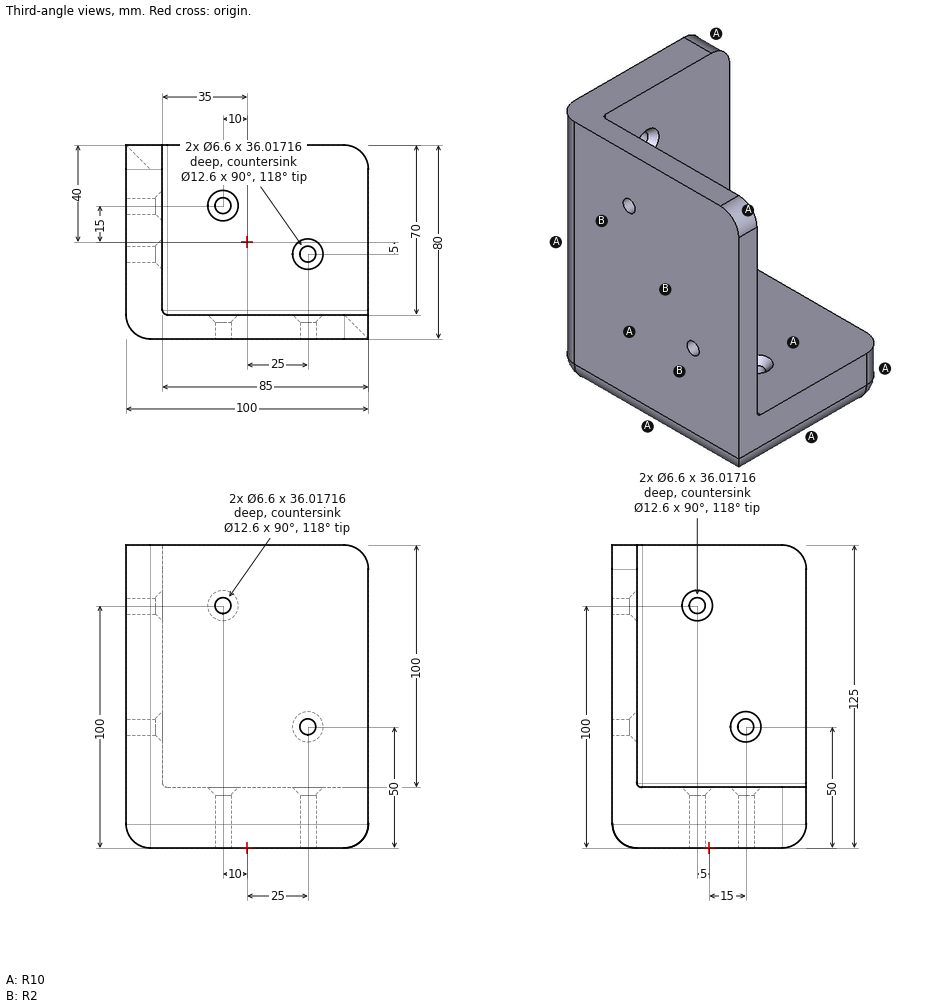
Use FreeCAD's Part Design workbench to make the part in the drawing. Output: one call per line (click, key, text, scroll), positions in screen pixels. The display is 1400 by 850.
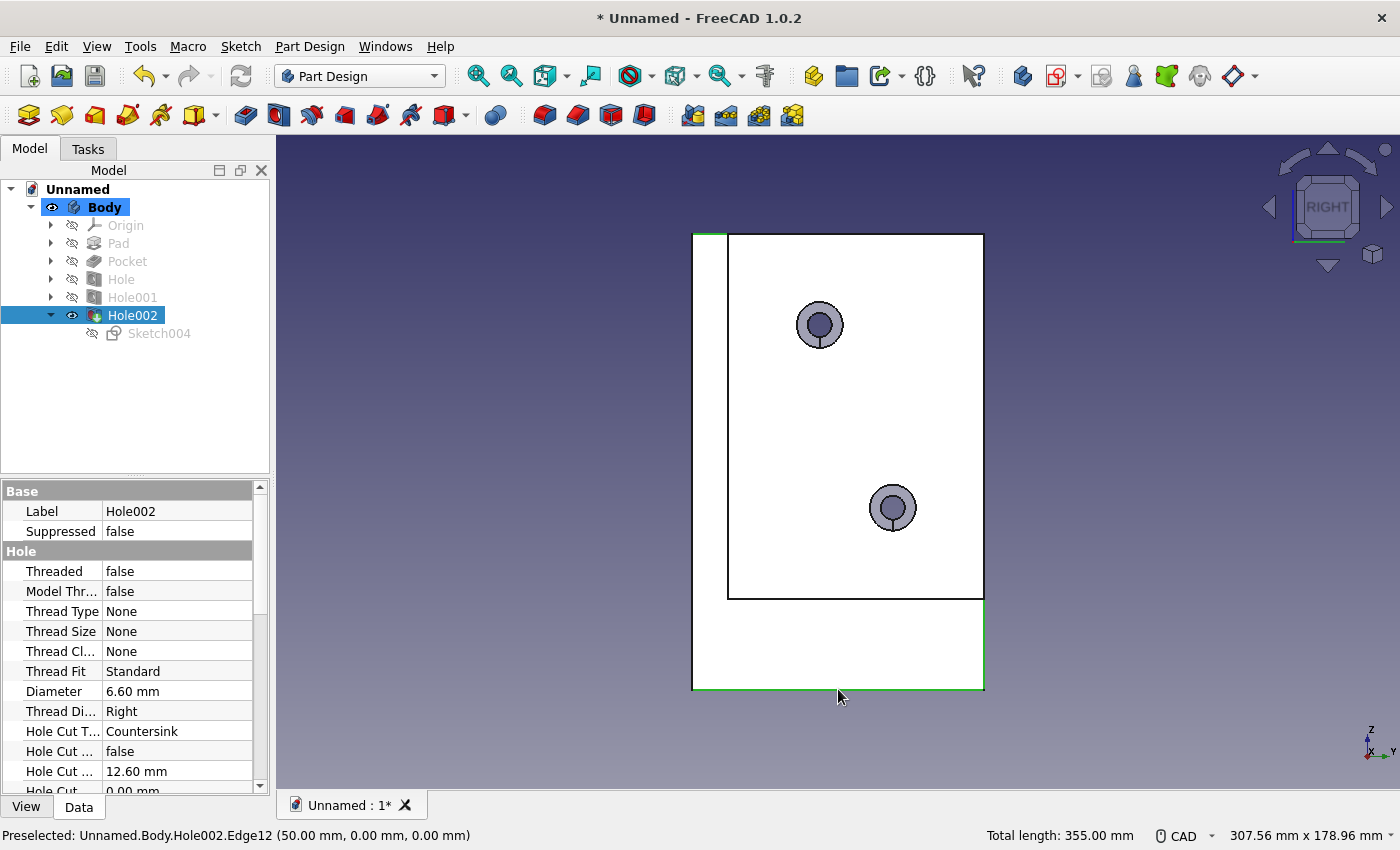
key(5)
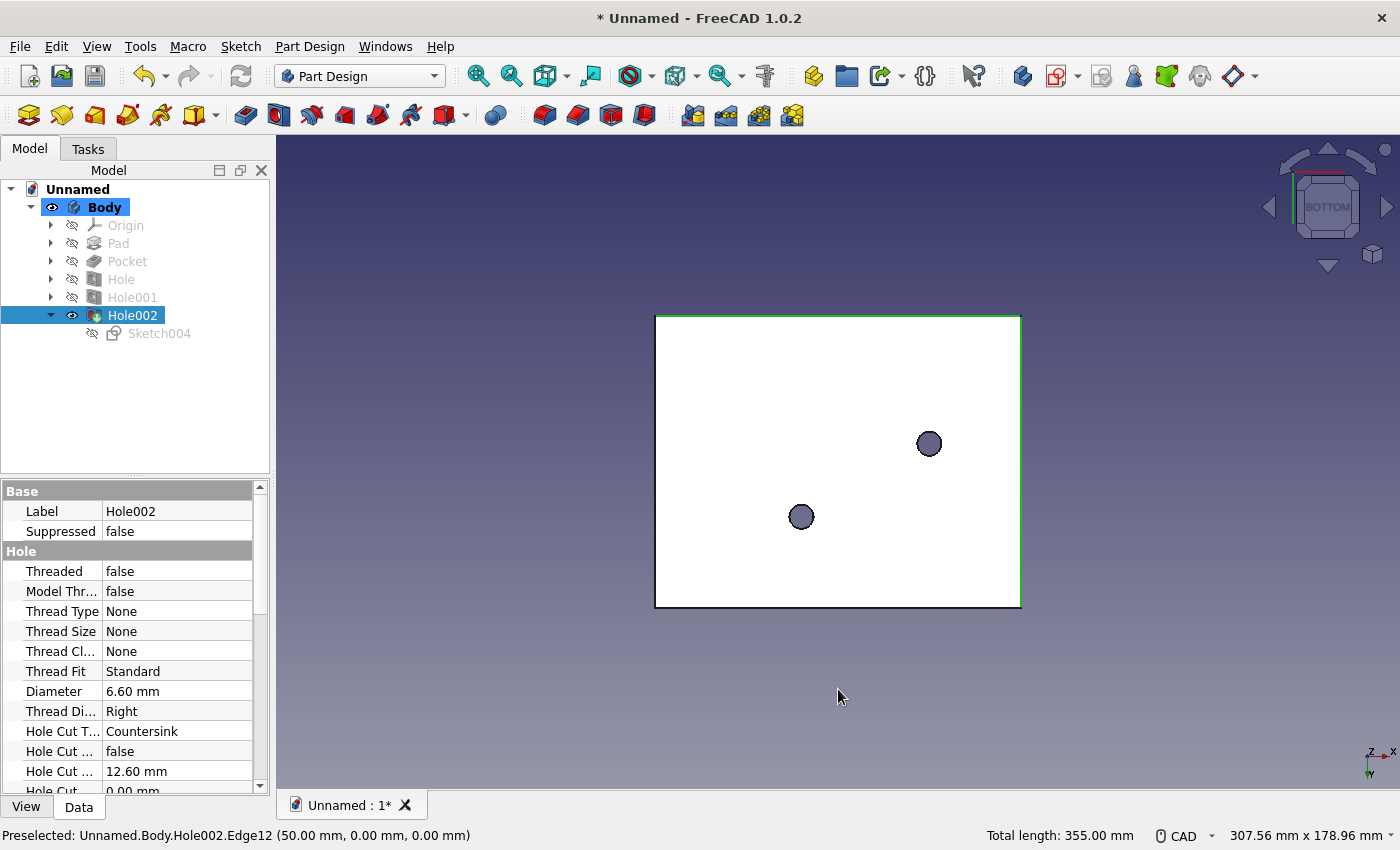
click(479, 76)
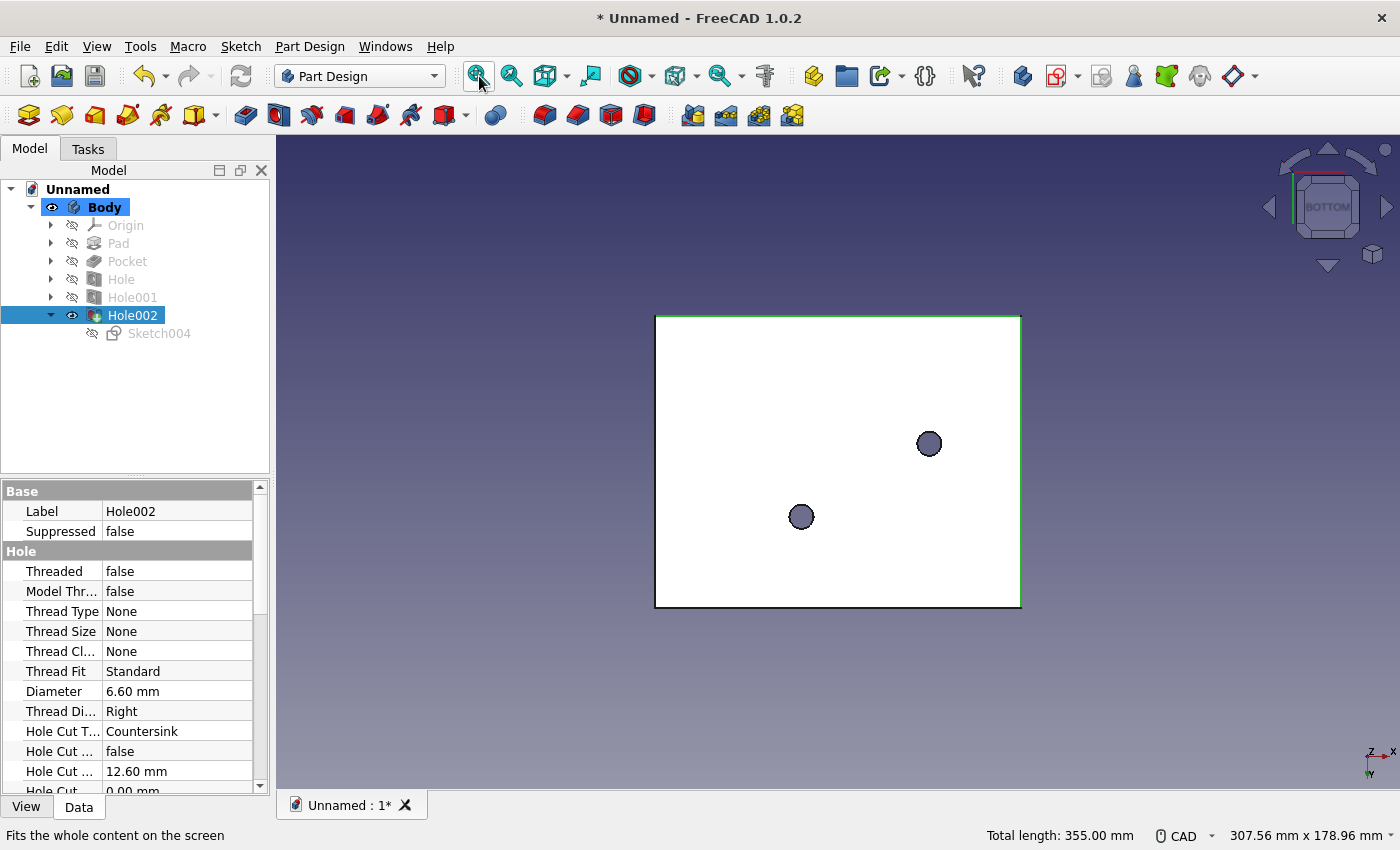
click(838, 607, ctrl)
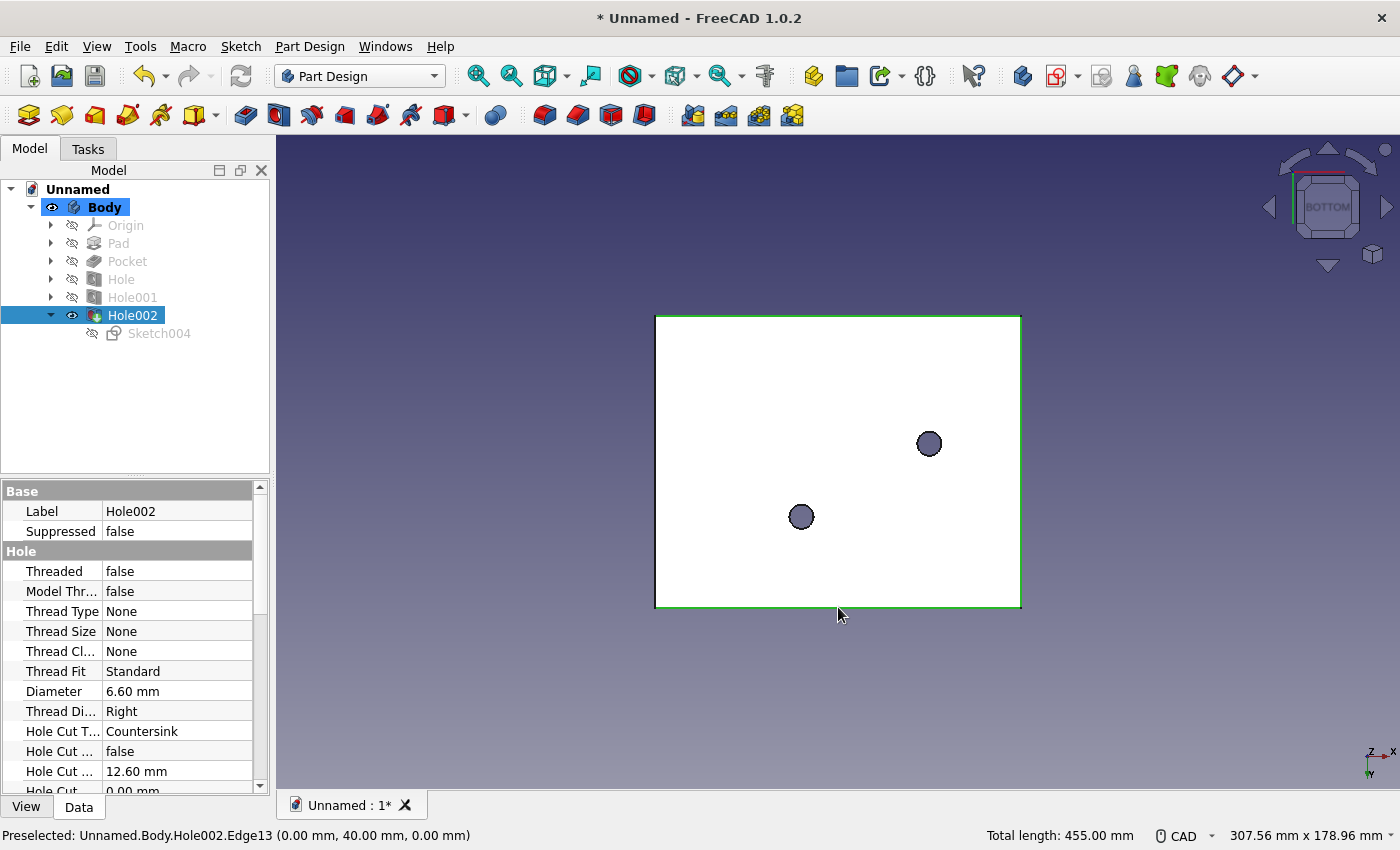
click(655, 461, ctrl)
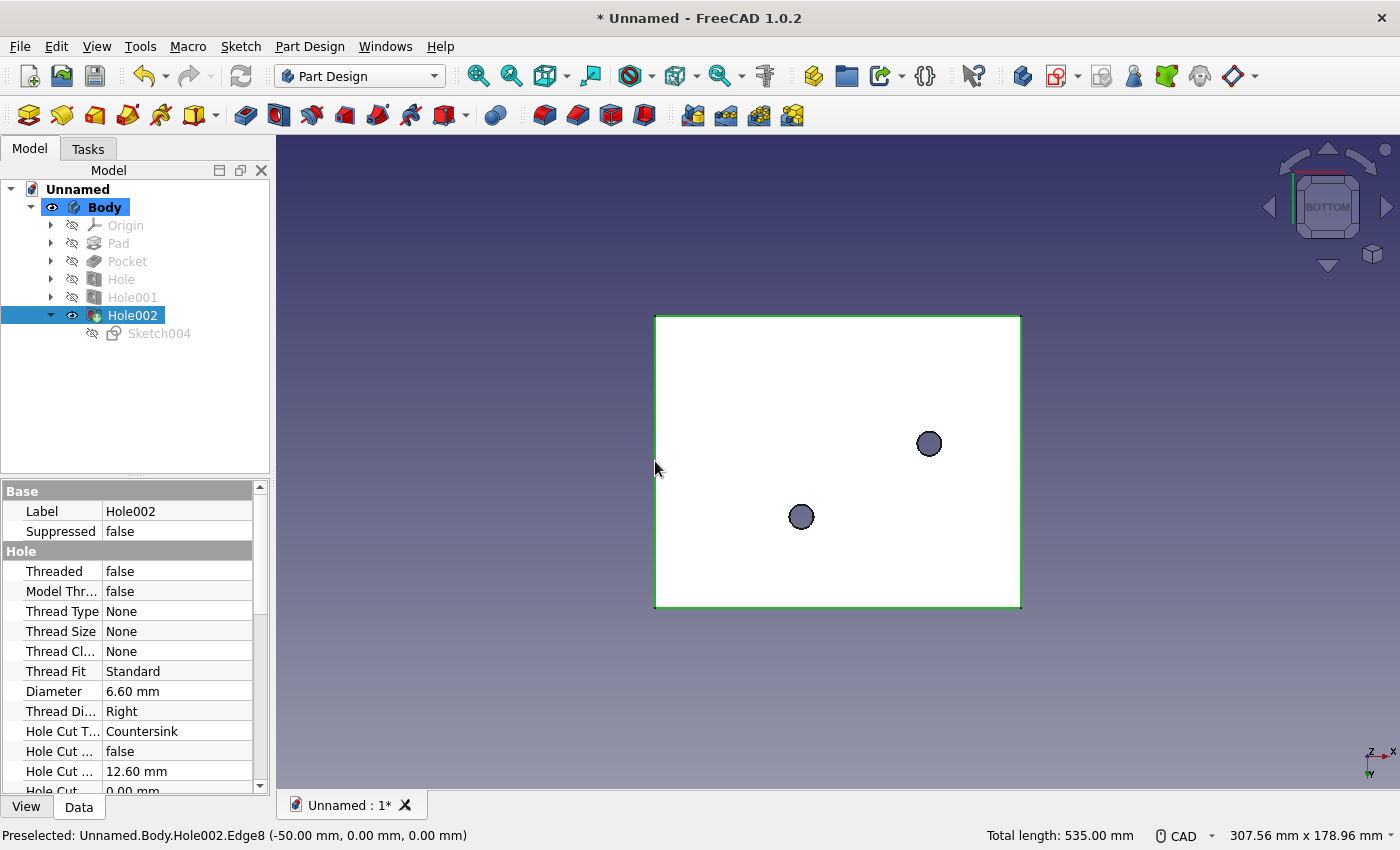
click(545, 116)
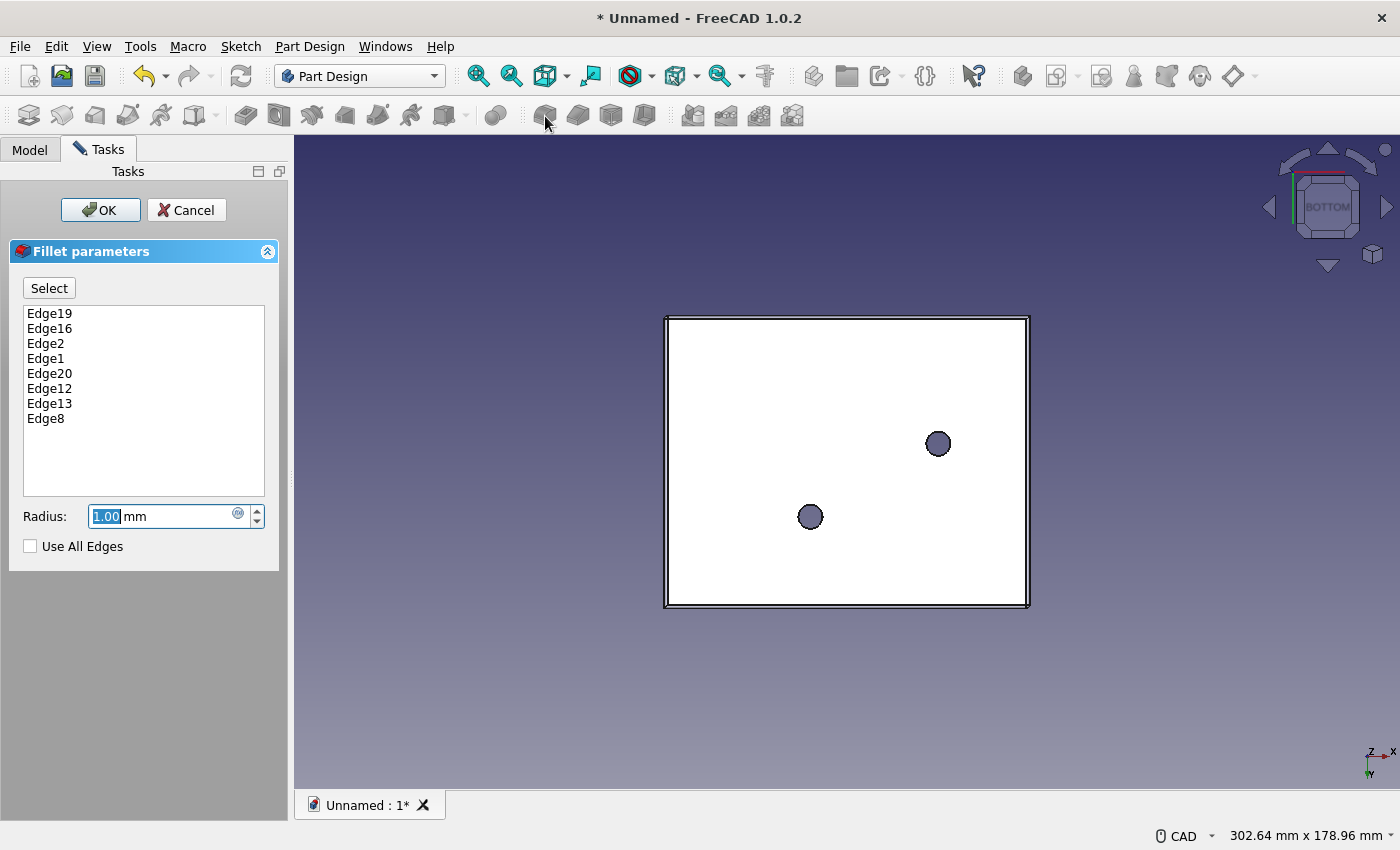
text(10)
key(Tab)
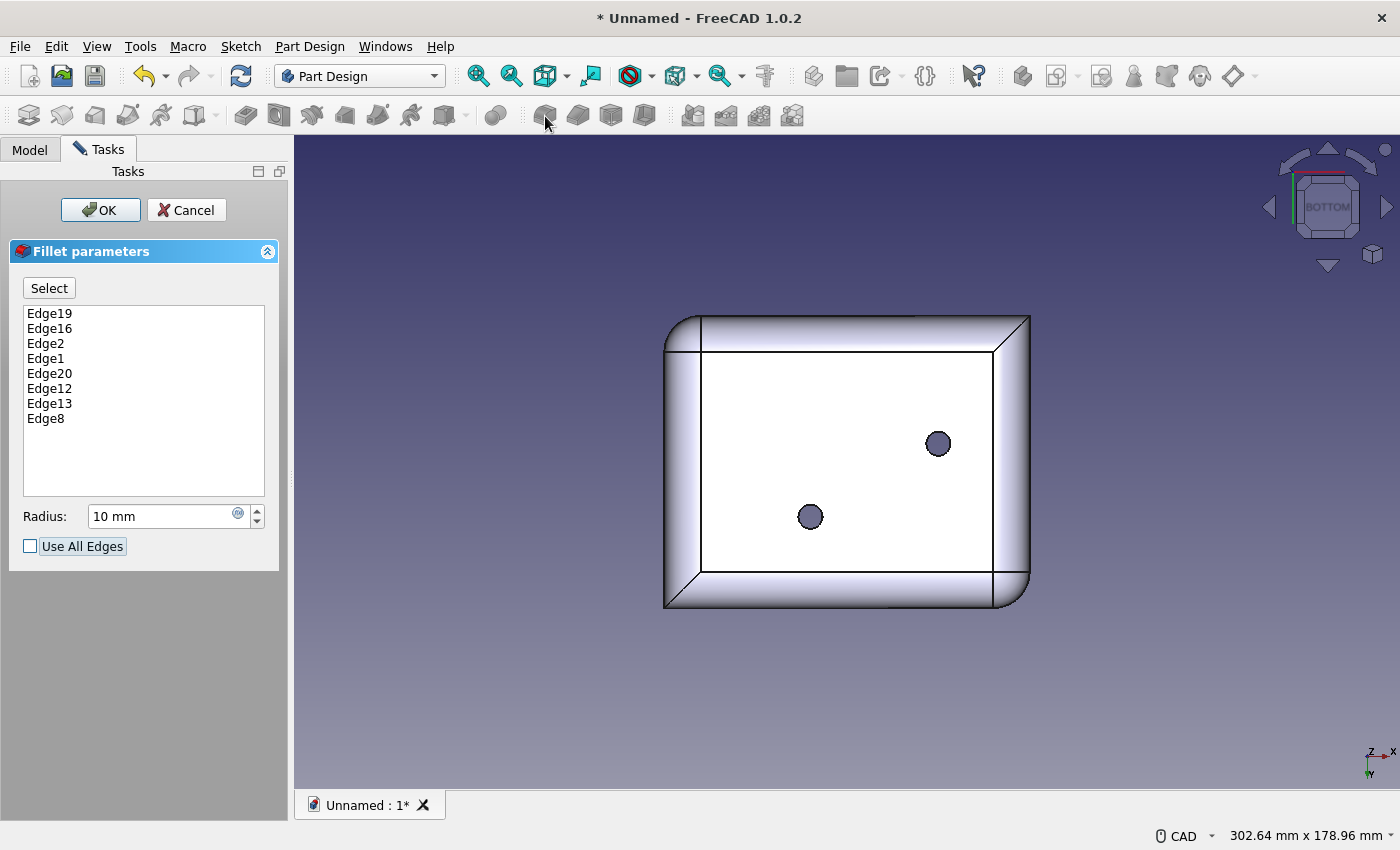
click(101, 210)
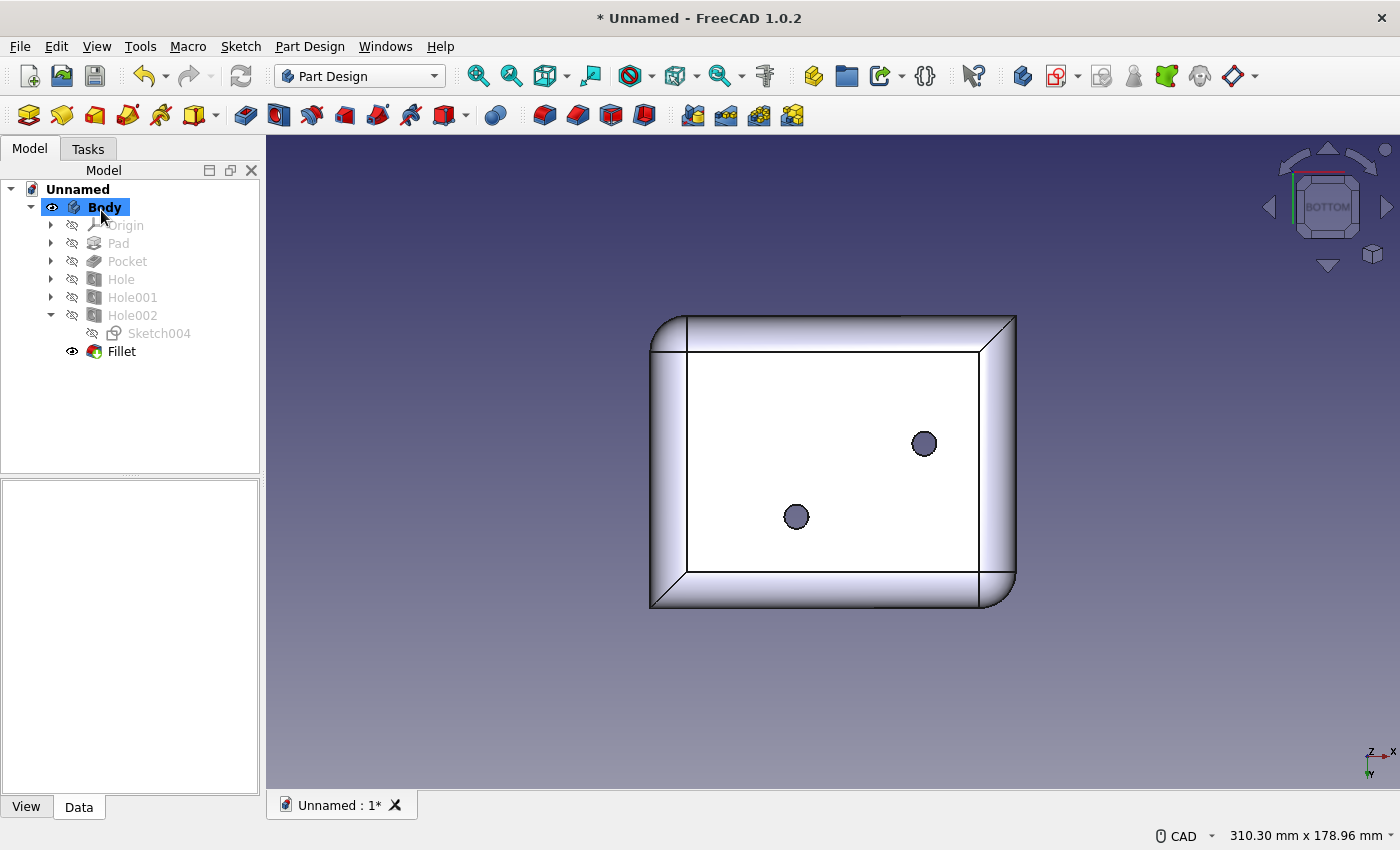
key(v)
key(f)